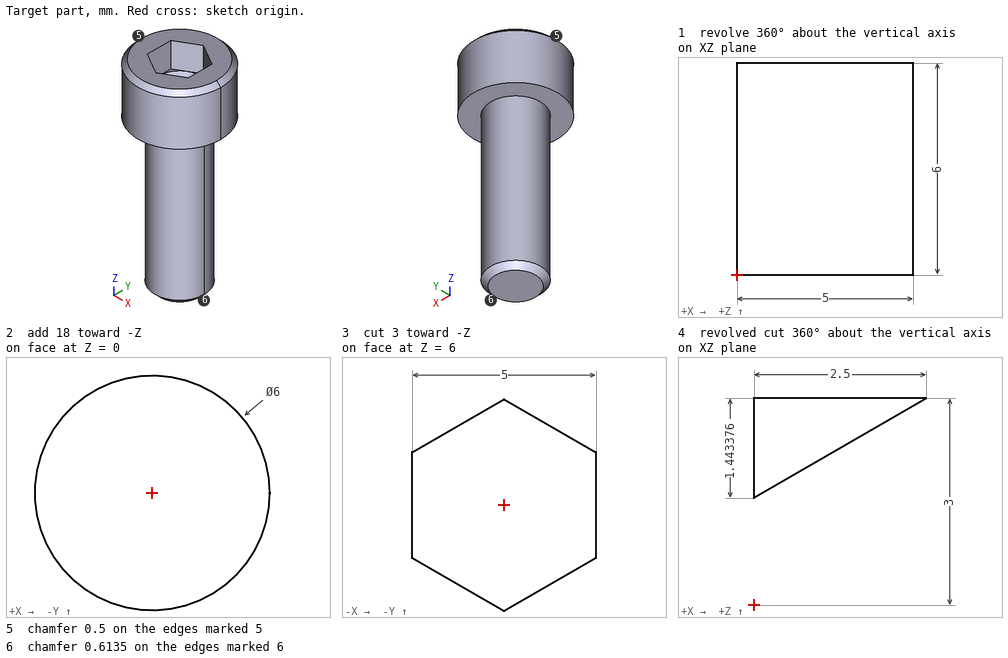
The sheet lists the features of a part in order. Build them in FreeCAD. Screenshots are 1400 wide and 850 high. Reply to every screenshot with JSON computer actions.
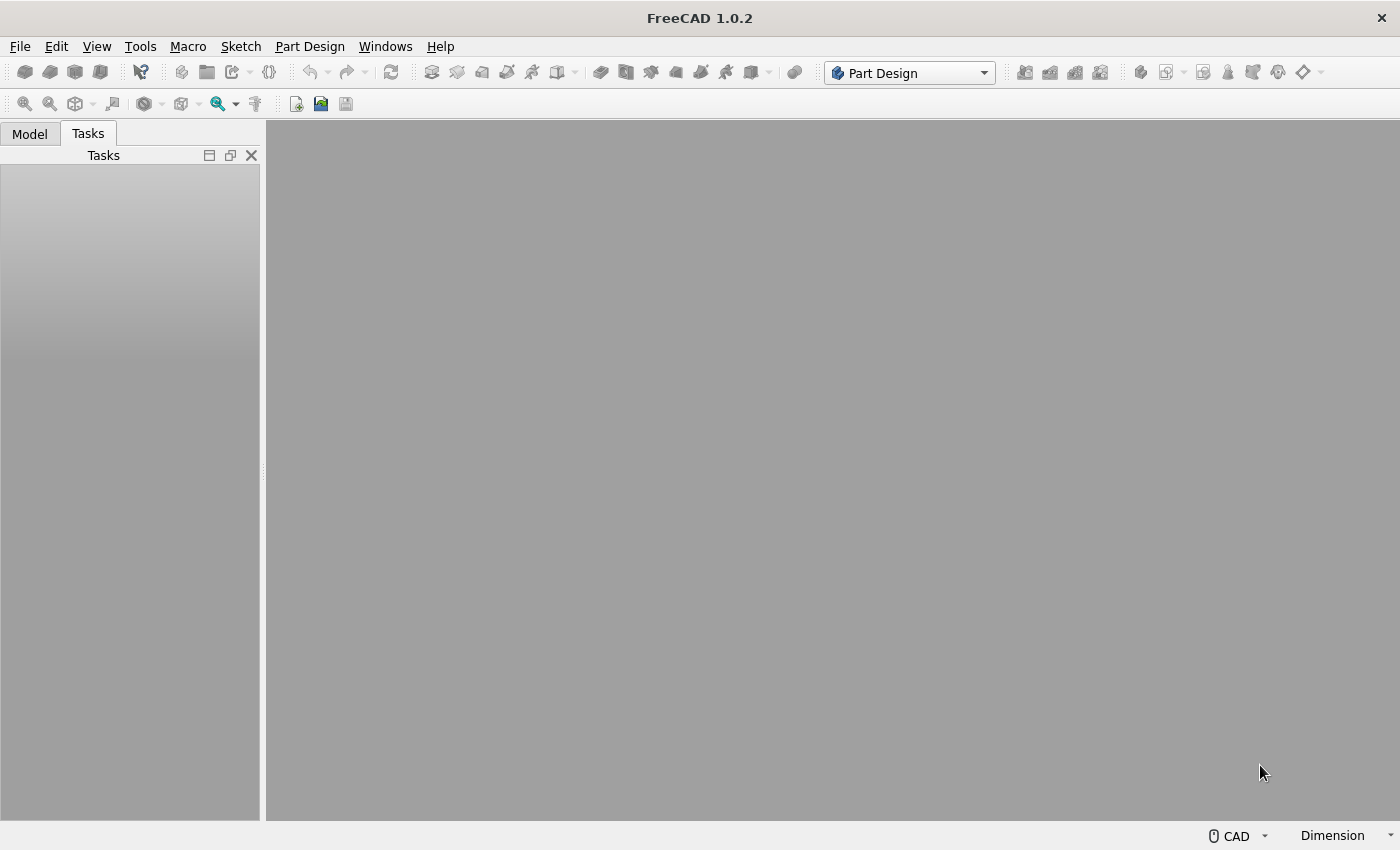
{"action": "left_click", "coordinate": [296, 104]}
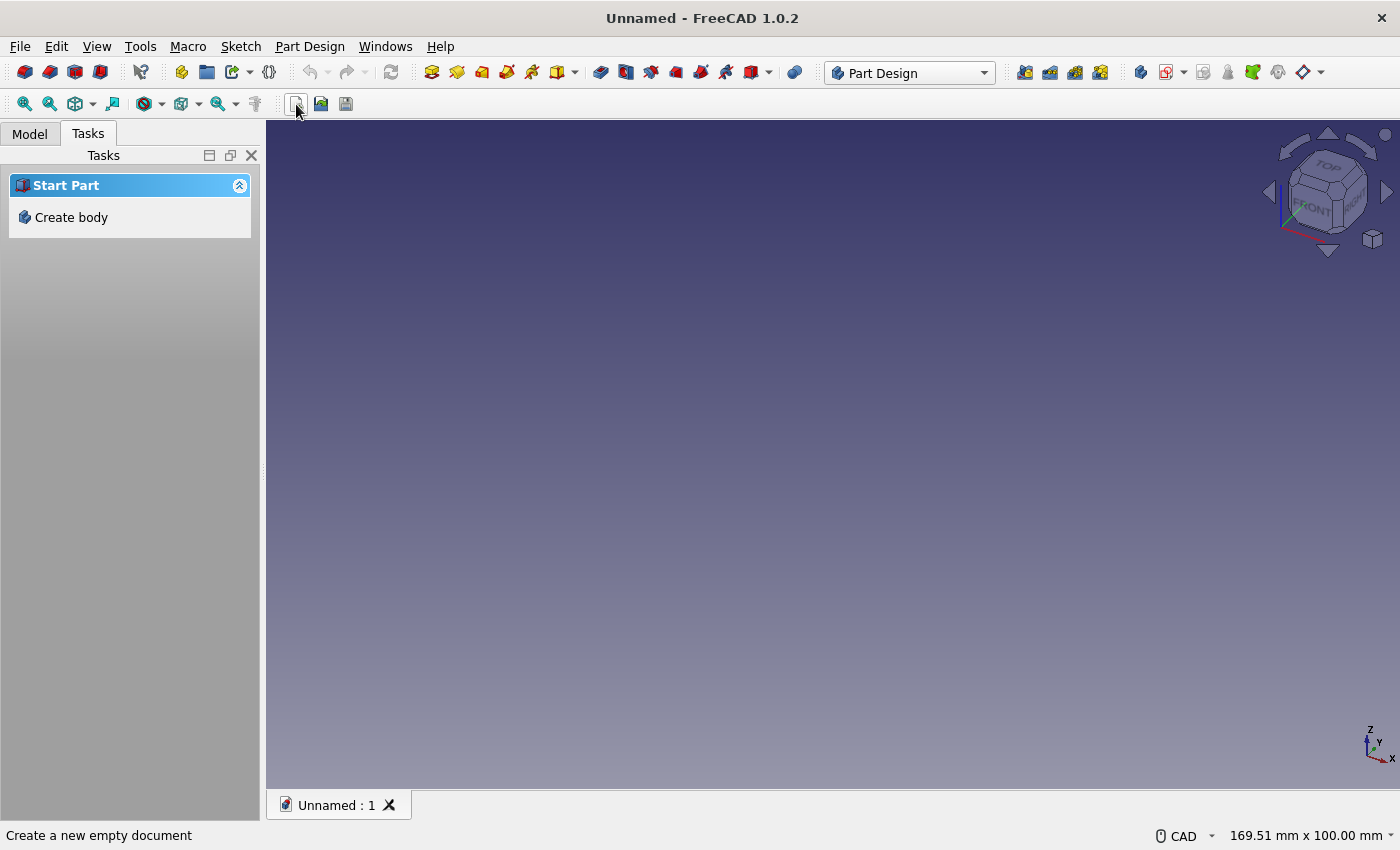
{"action": "left_click", "coordinate": [1166, 72]}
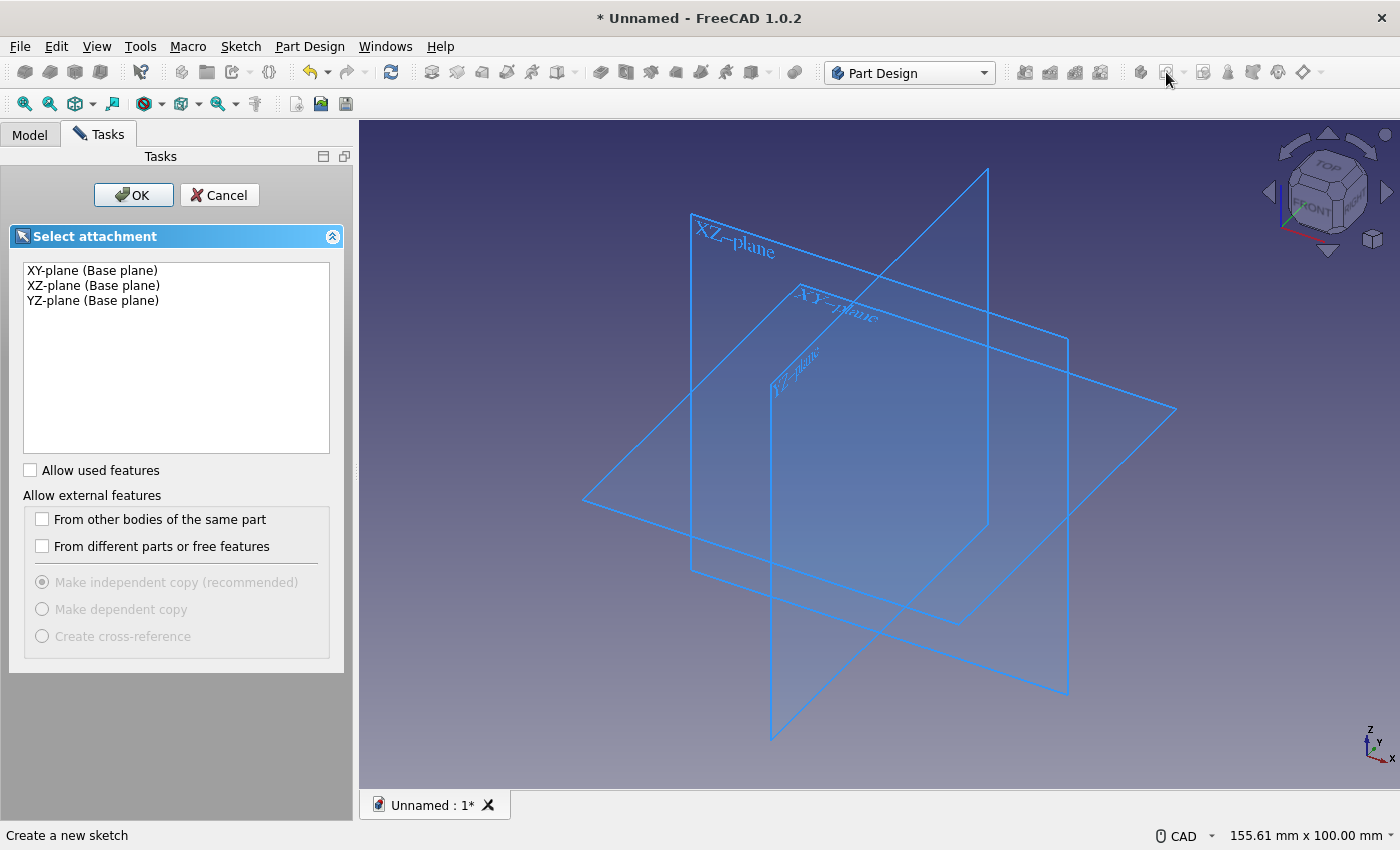
{"action": "left_click", "coordinate": [84, 286]}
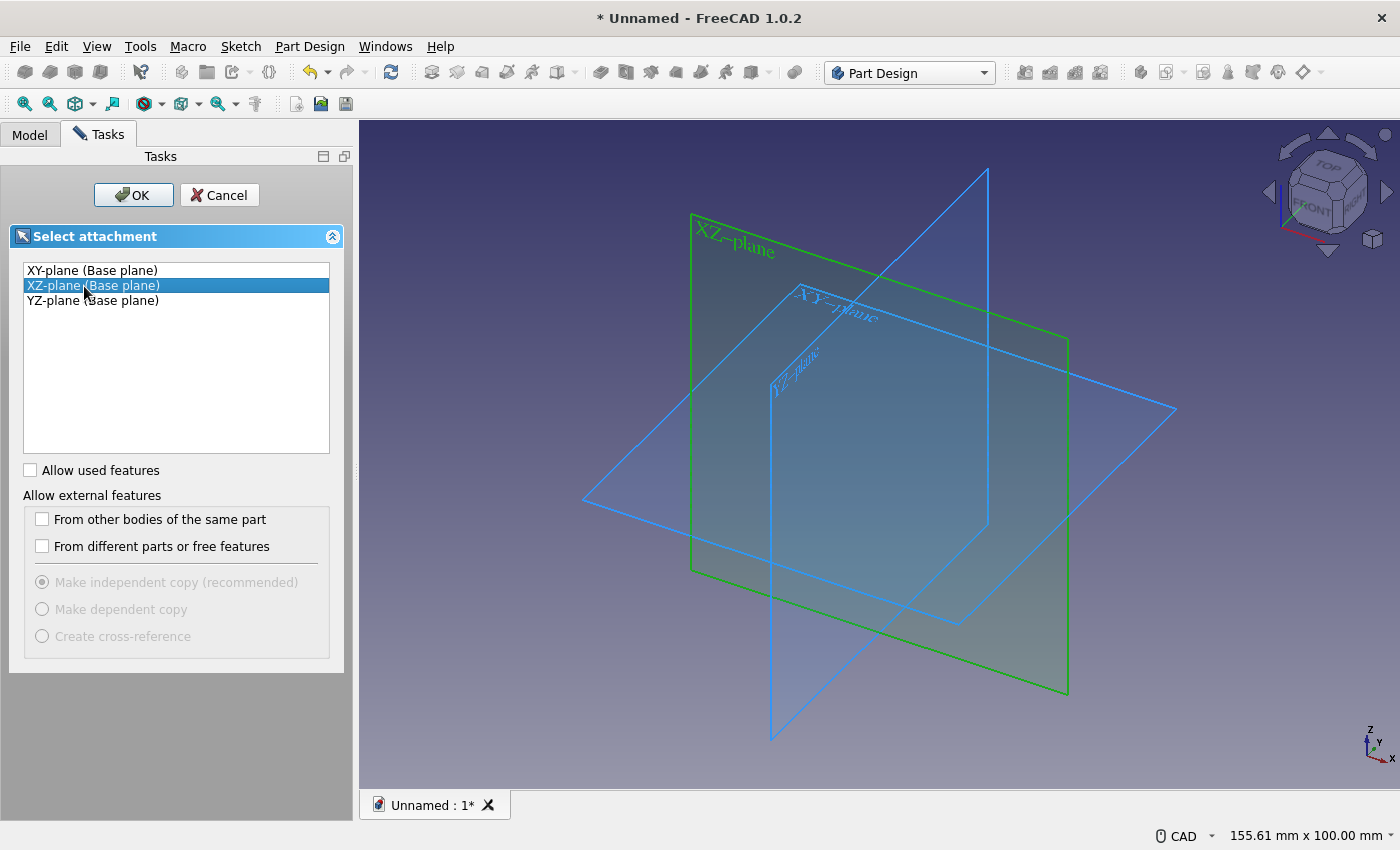
{"action": "left_click", "coordinate": [134, 195]}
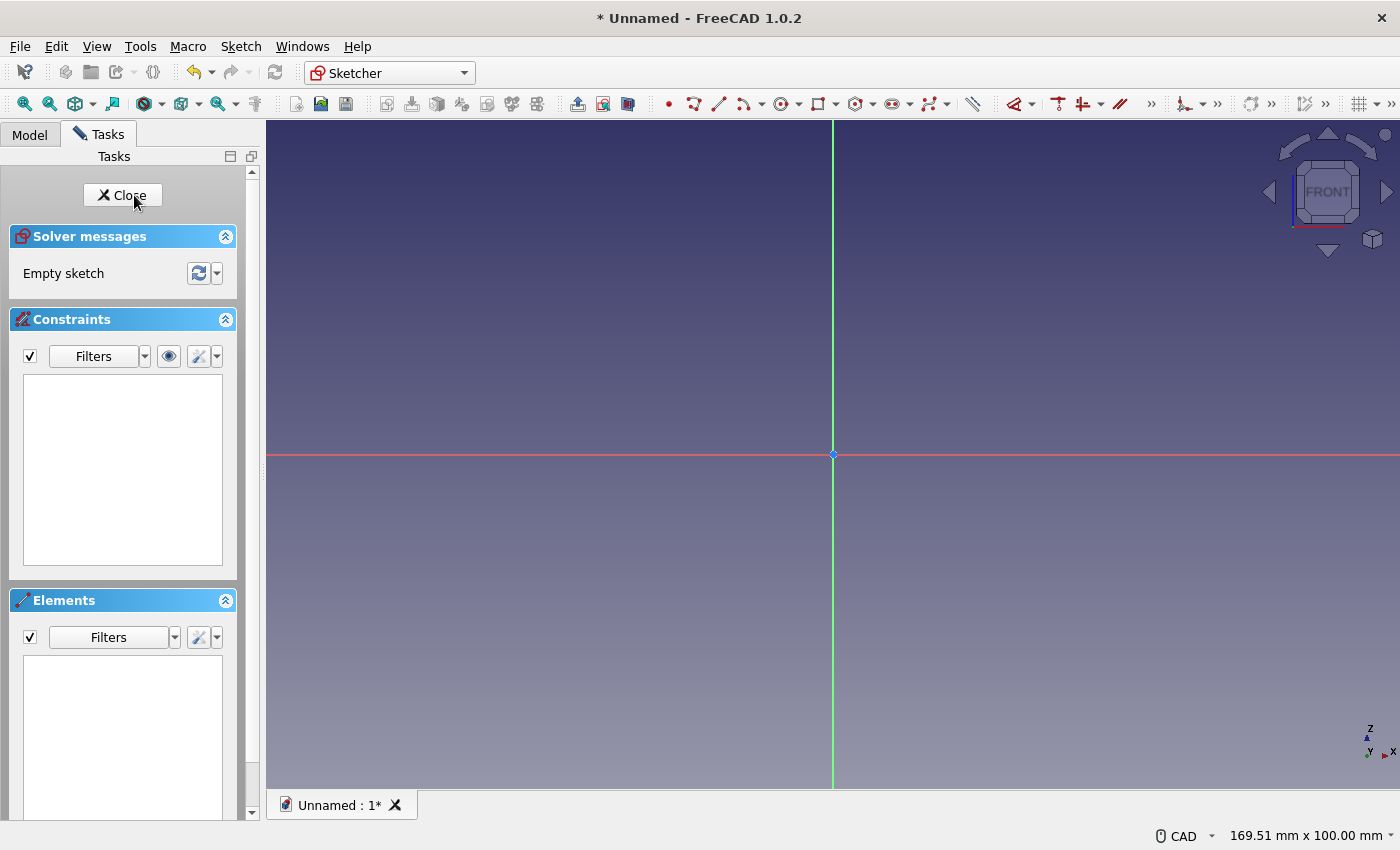
{"action": "scroll", "coordinate": [858, 432], "scroll_direction": "up", "scroll_amount": 12}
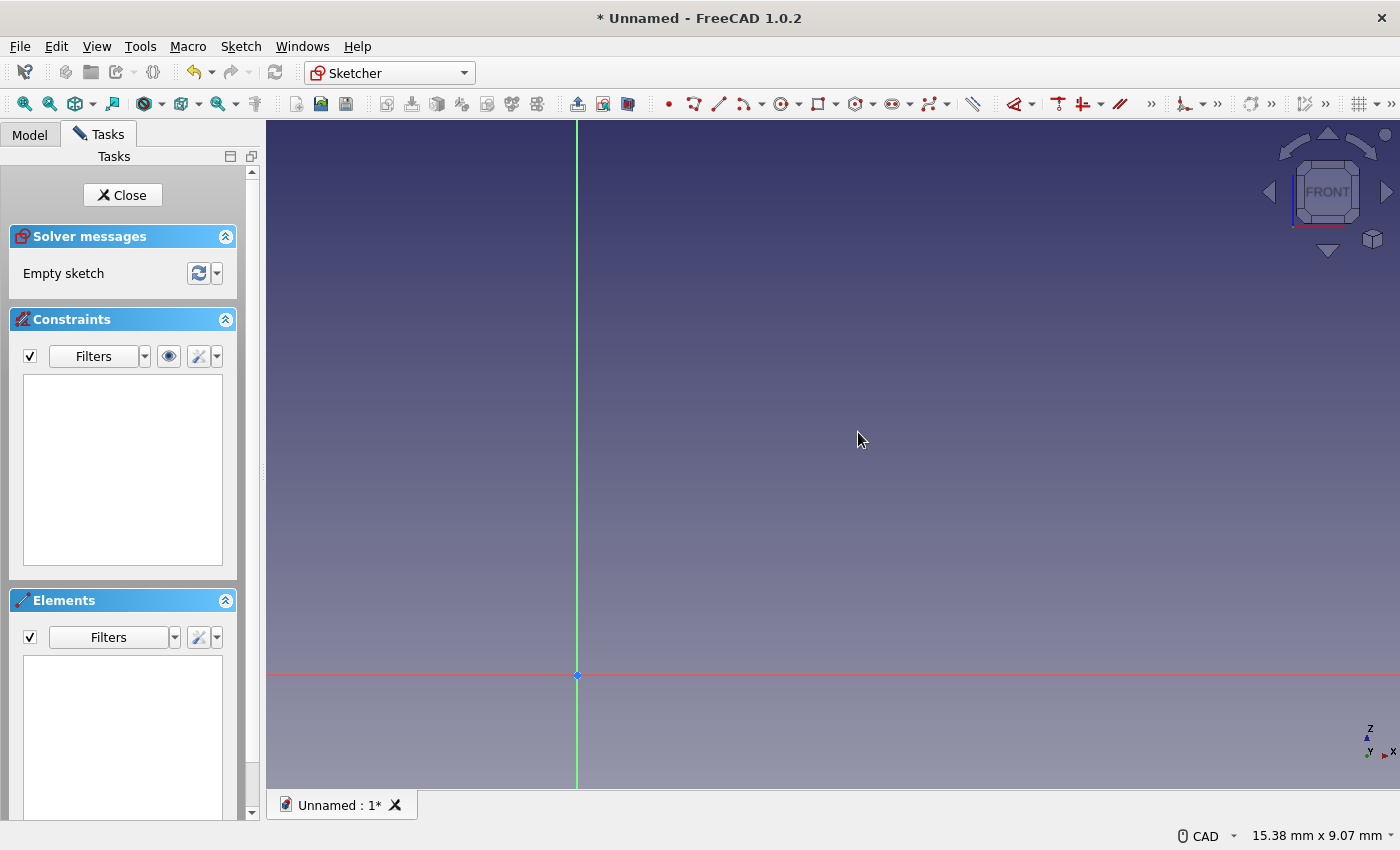
{"action": "left_click", "coordinate": [818, 104]}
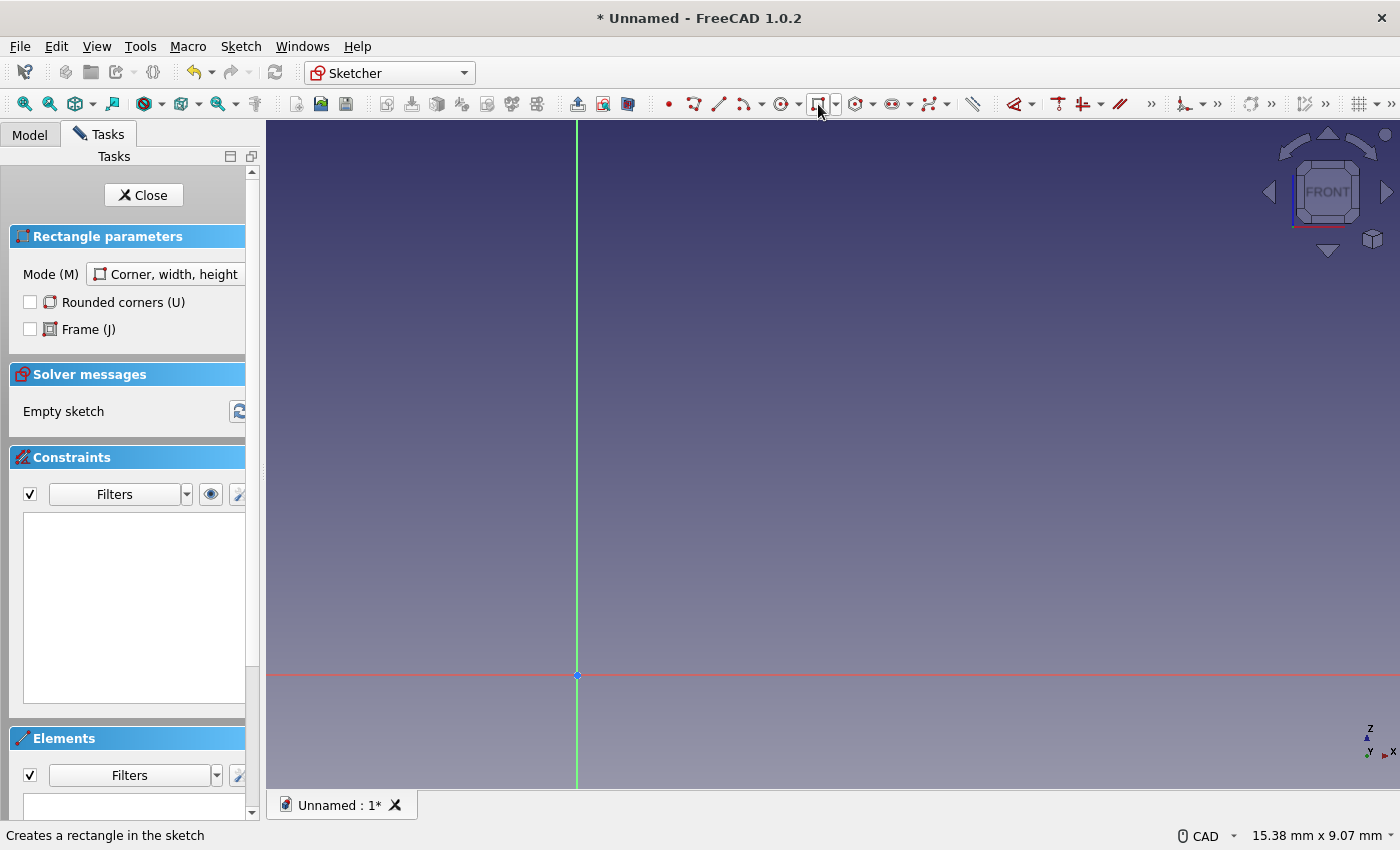
{"action": "left_click", "coordinate": [577, 675]}
{"action": "mouse_move", "coordinate": [946, 233]}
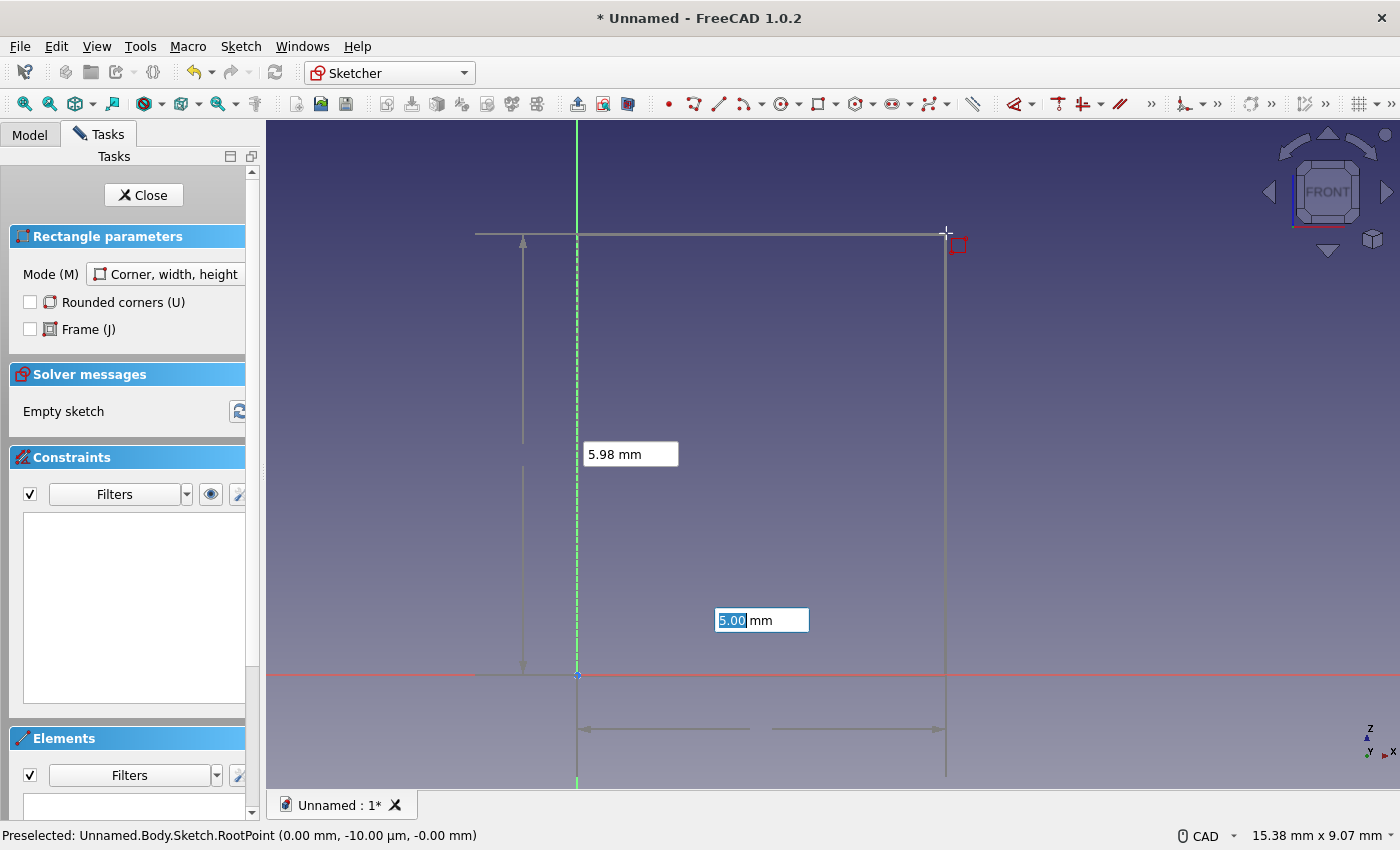
{"action": "type", "text": "5"}
{"action": "key", "text": "Tab"}
{"action": "type", "text": "6"}
{"action": "key", "text": "Return"}
{"action": "key", "text": "Escape"}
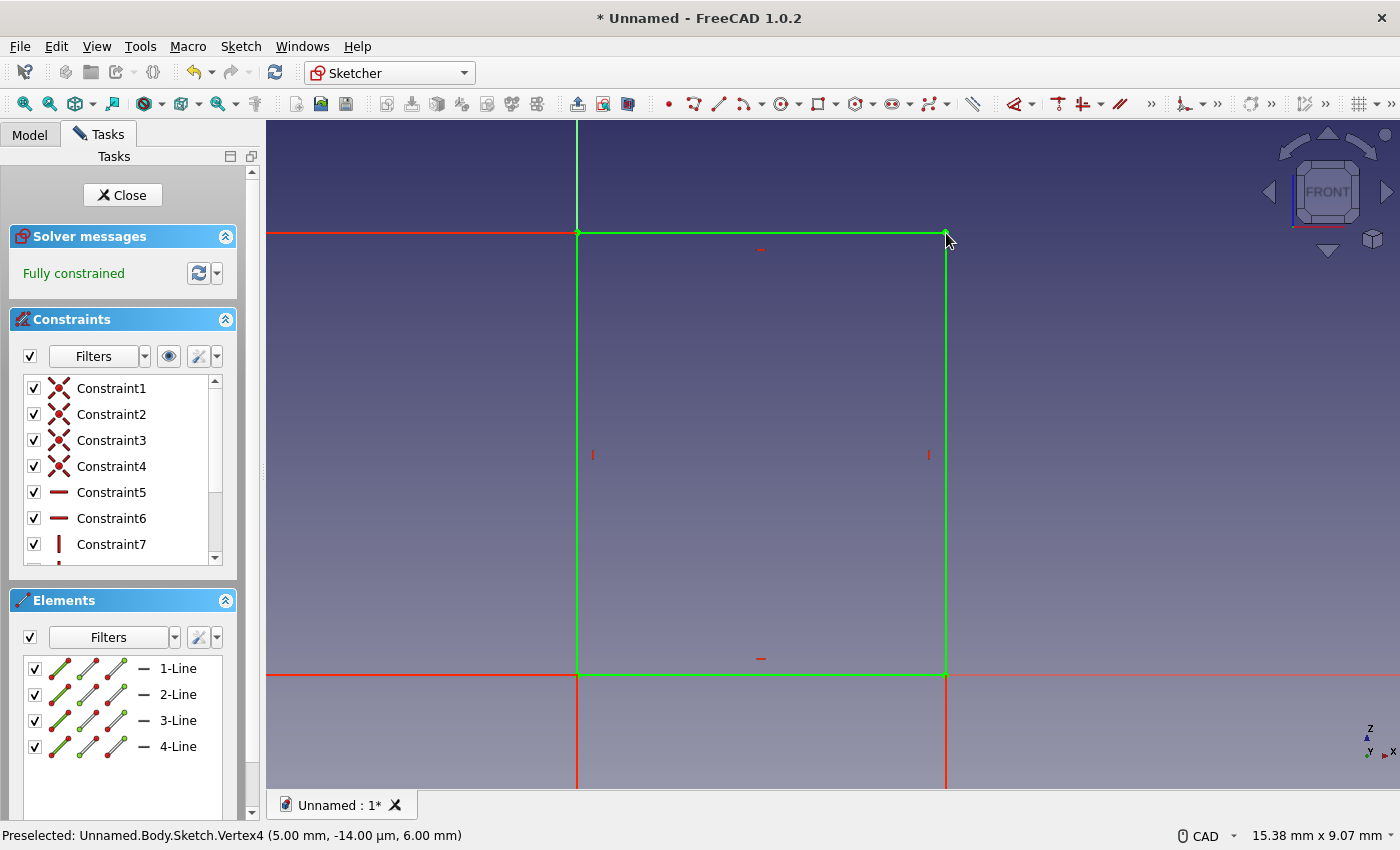
{"action": "left_click", "coordinate": [123, 195]}